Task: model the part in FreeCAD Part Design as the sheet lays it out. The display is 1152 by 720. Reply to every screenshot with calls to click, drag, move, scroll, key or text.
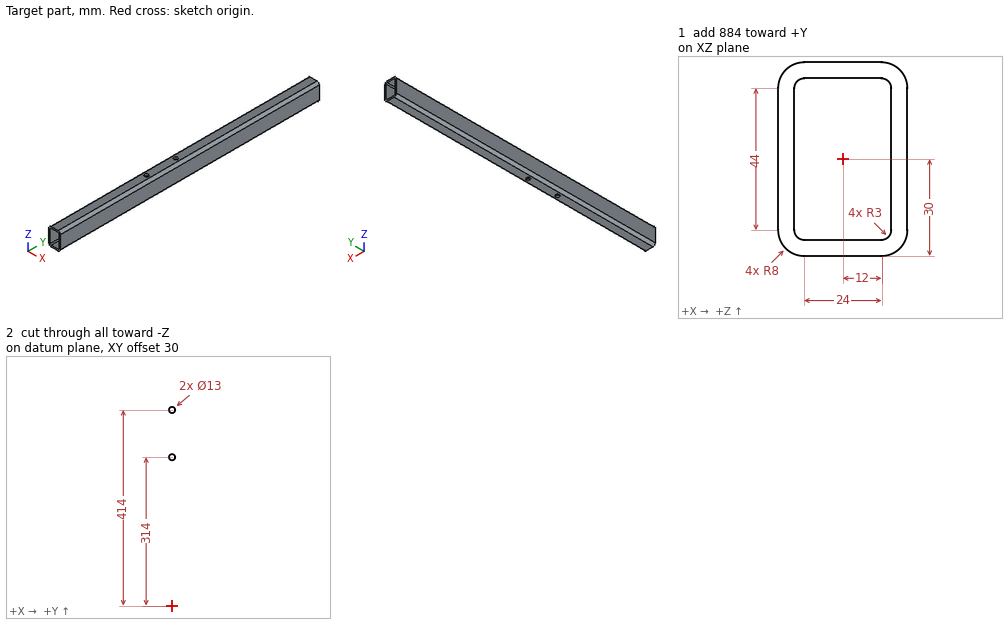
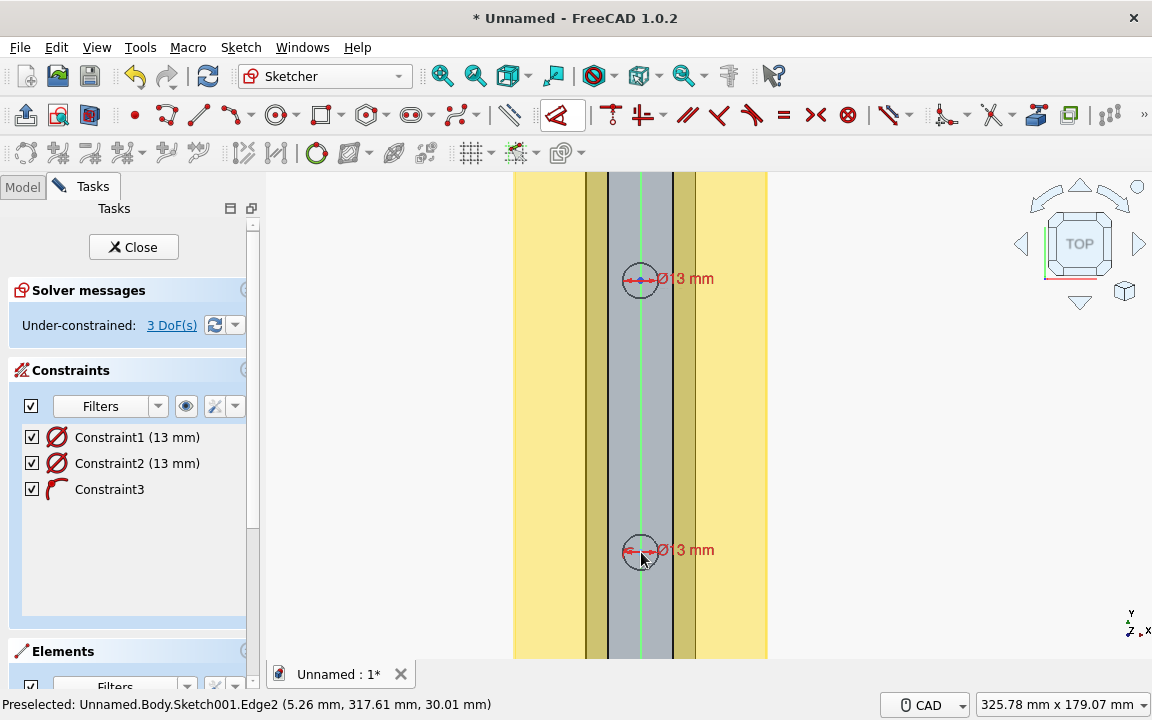
click(640, 281)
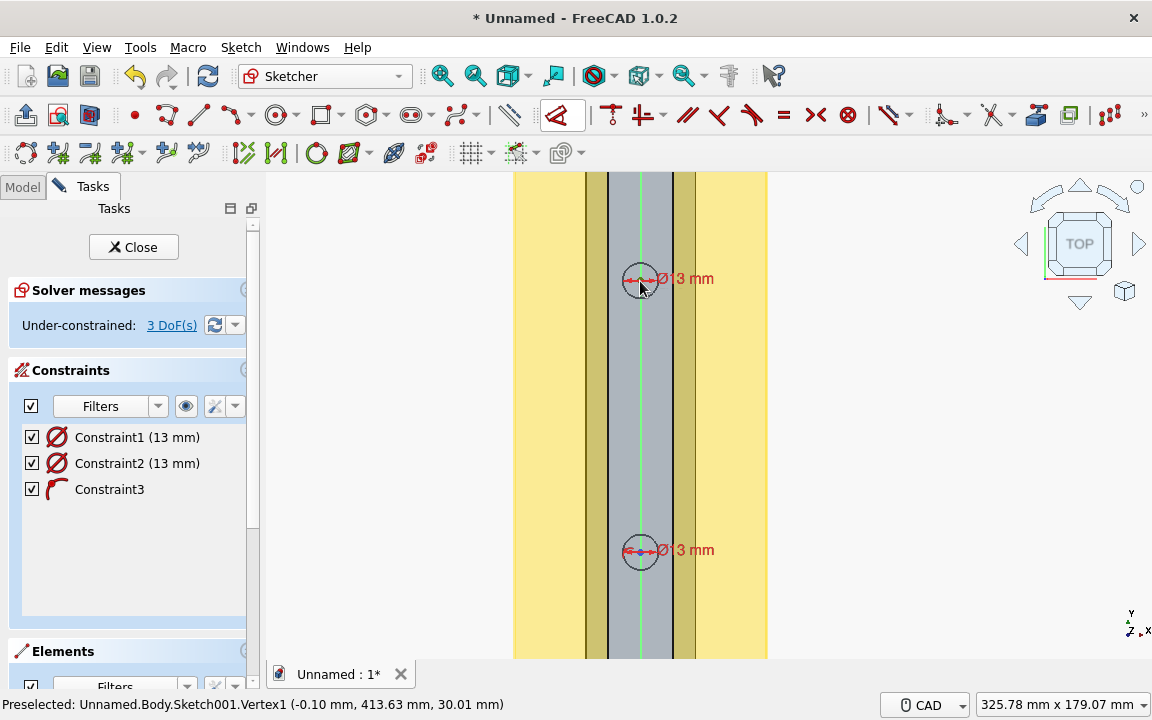
click(641, 600)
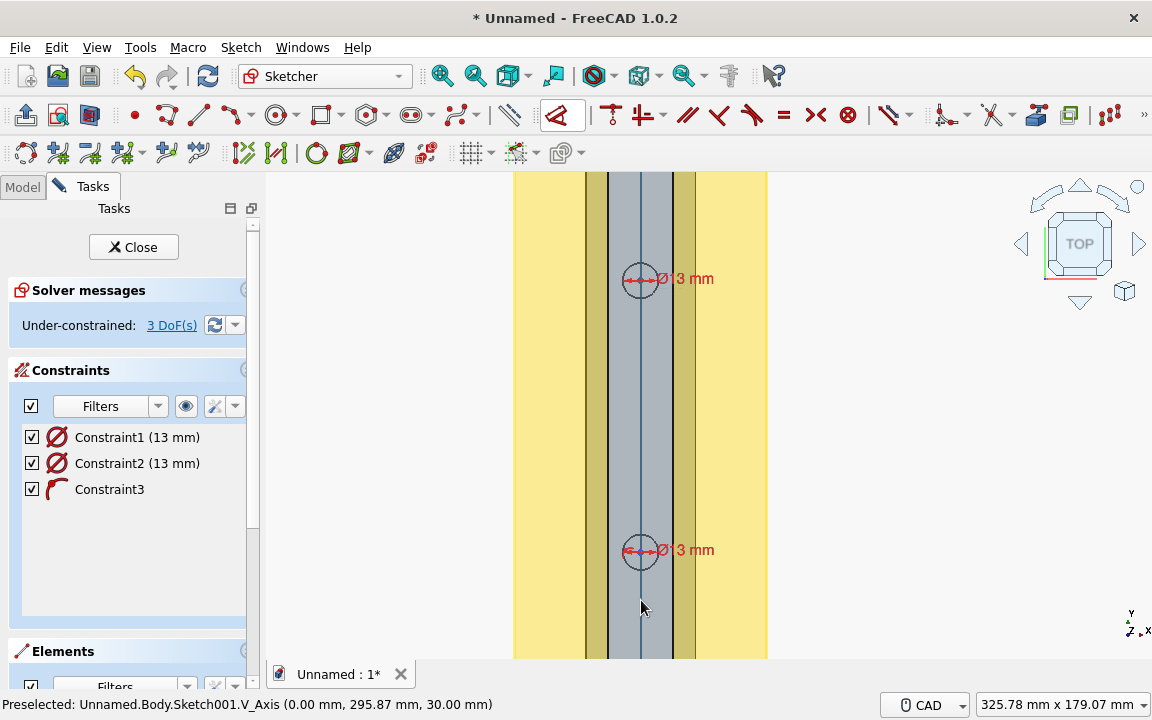
key(c)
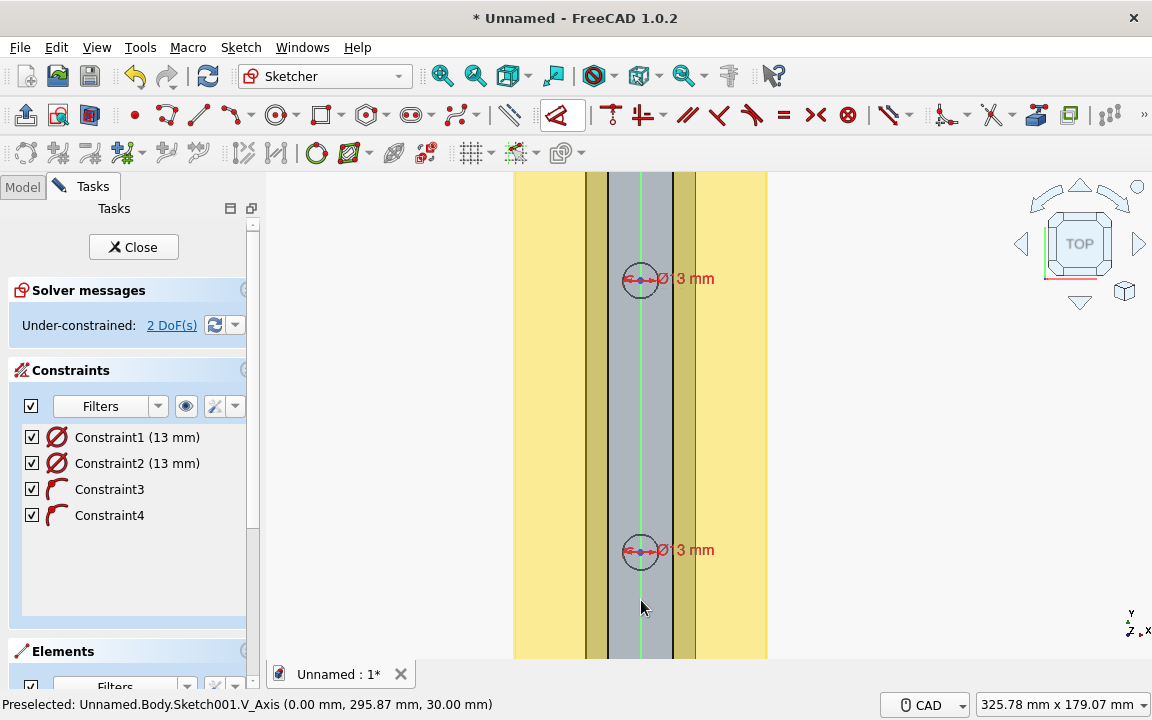
click(641, 281)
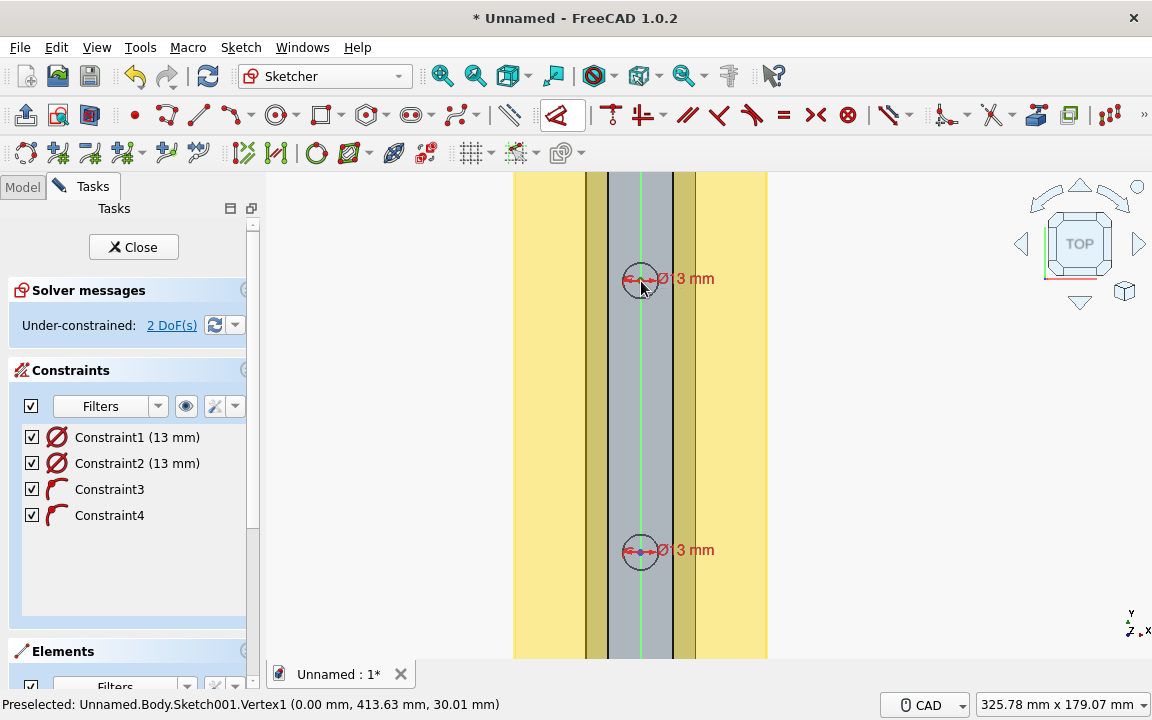
key(i)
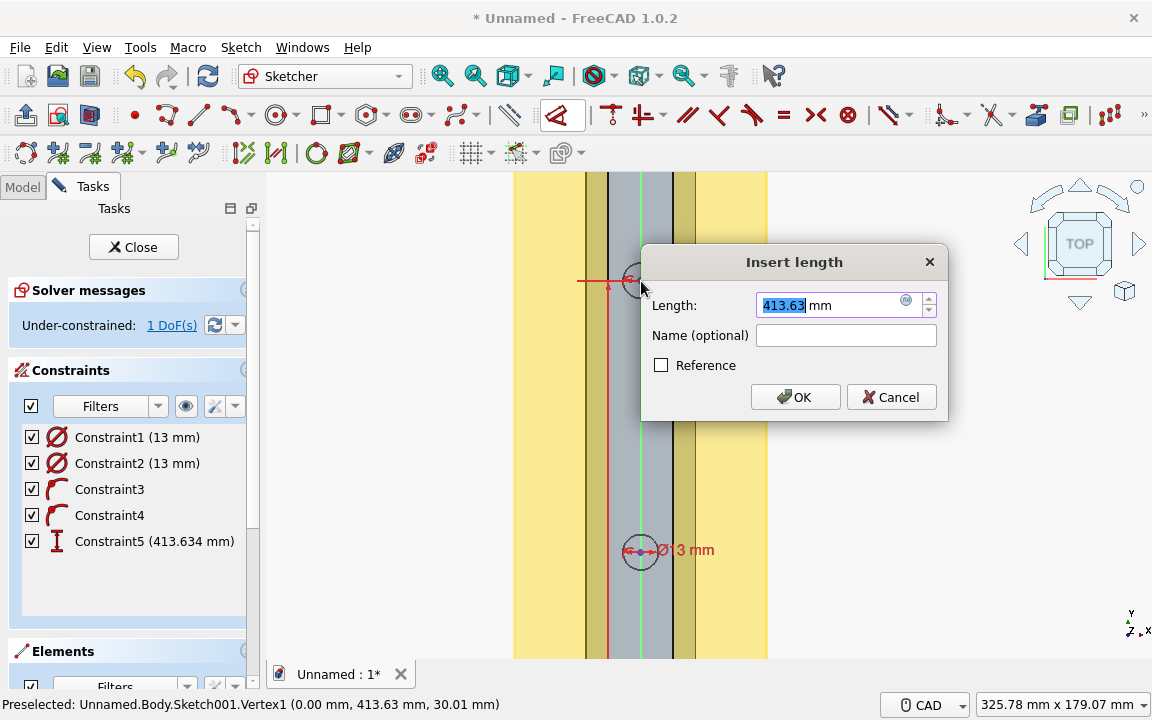
text(414)
key(Return)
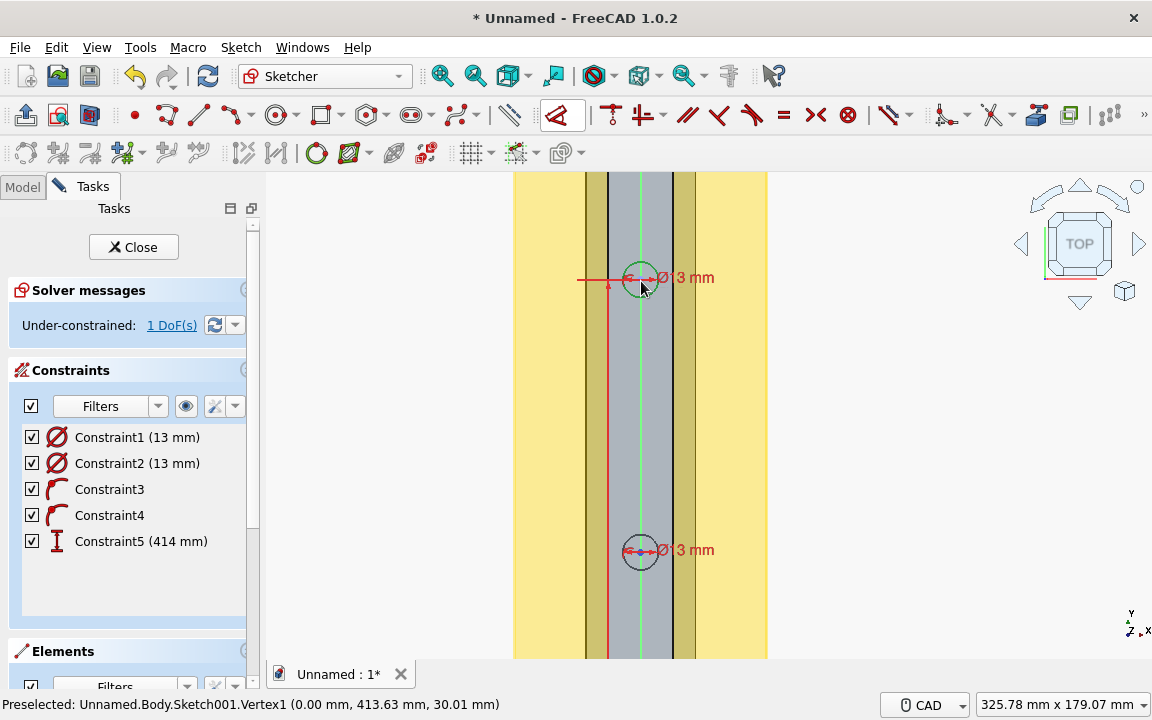
click(641, 552)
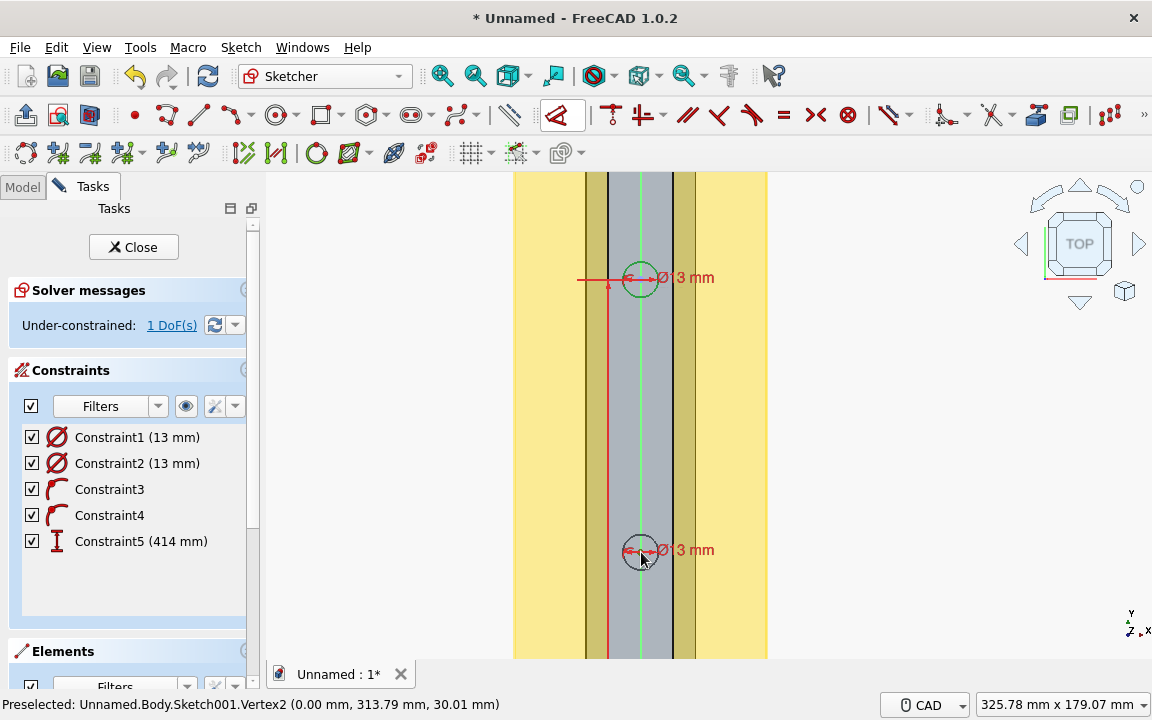
key(i)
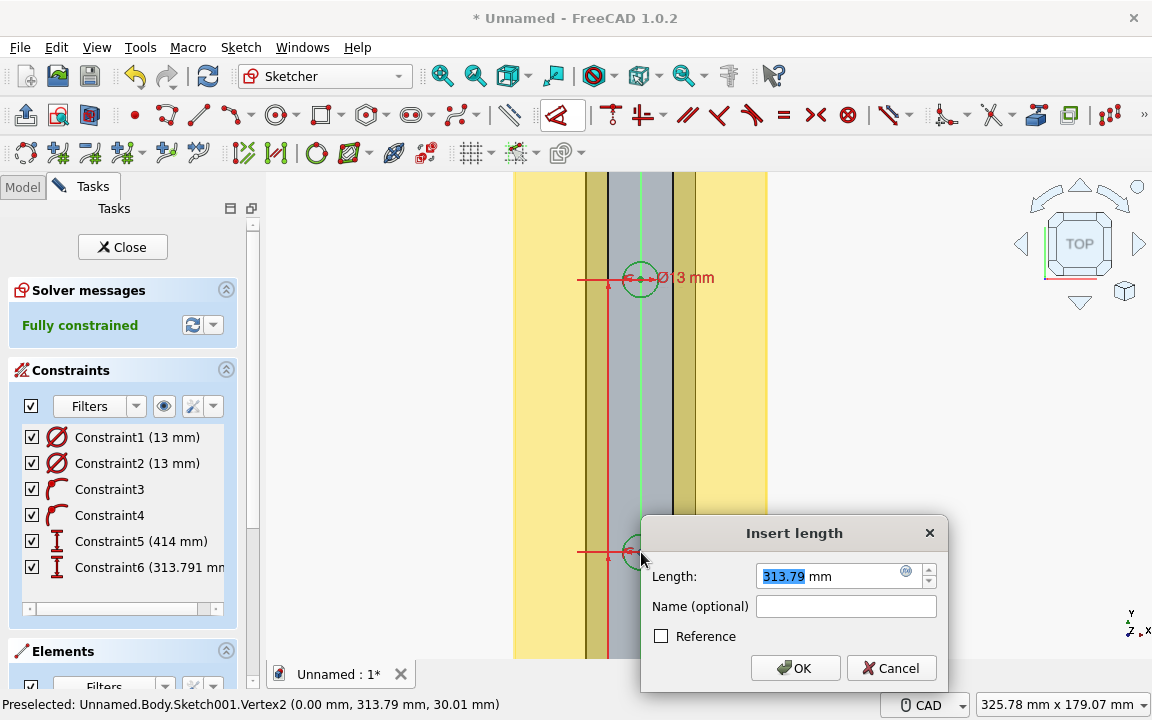
text(314)
key(Return)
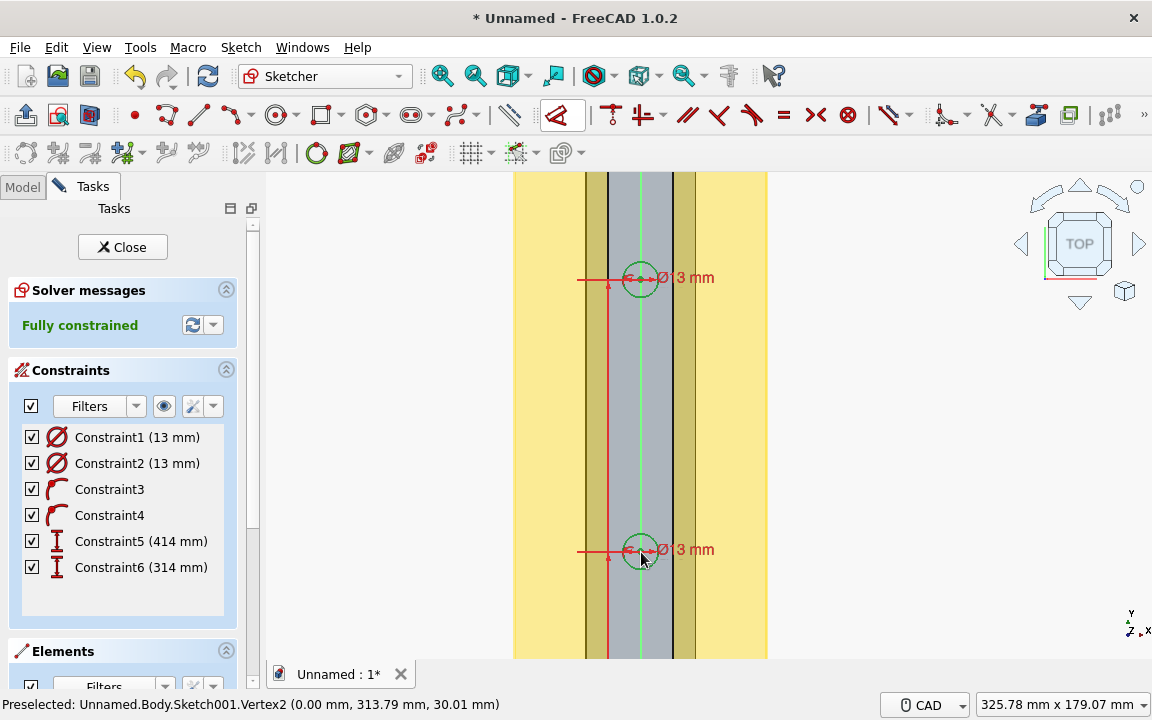
click(123, 247)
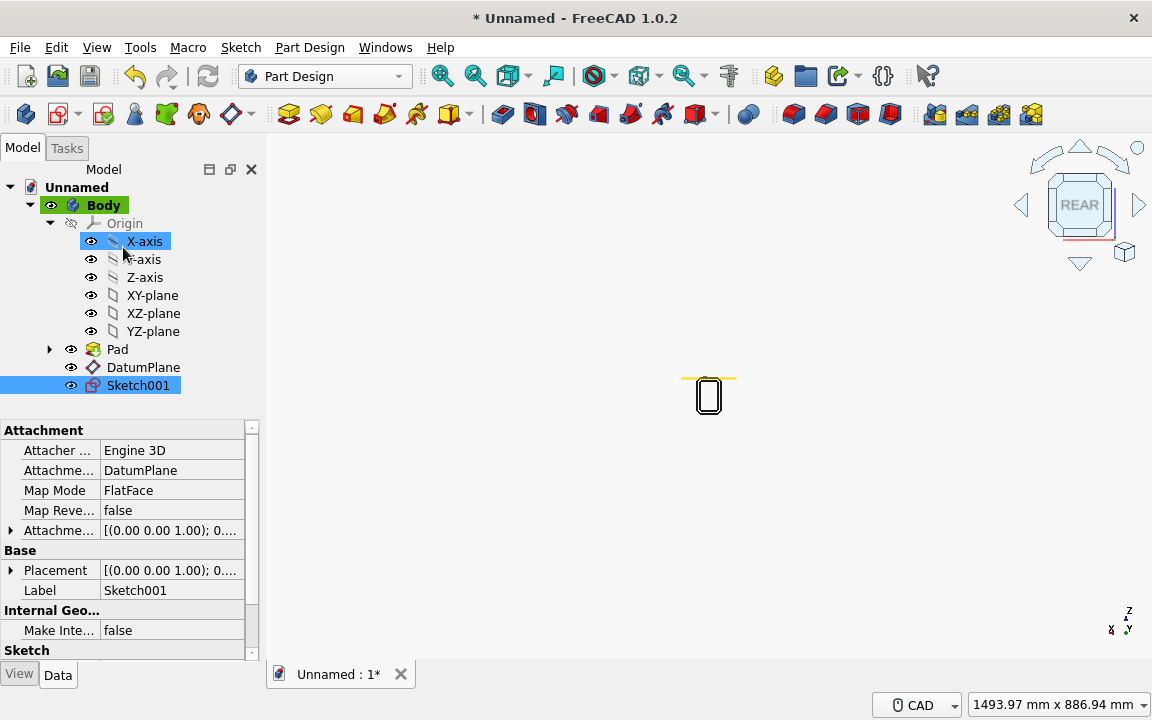
click(504, 114)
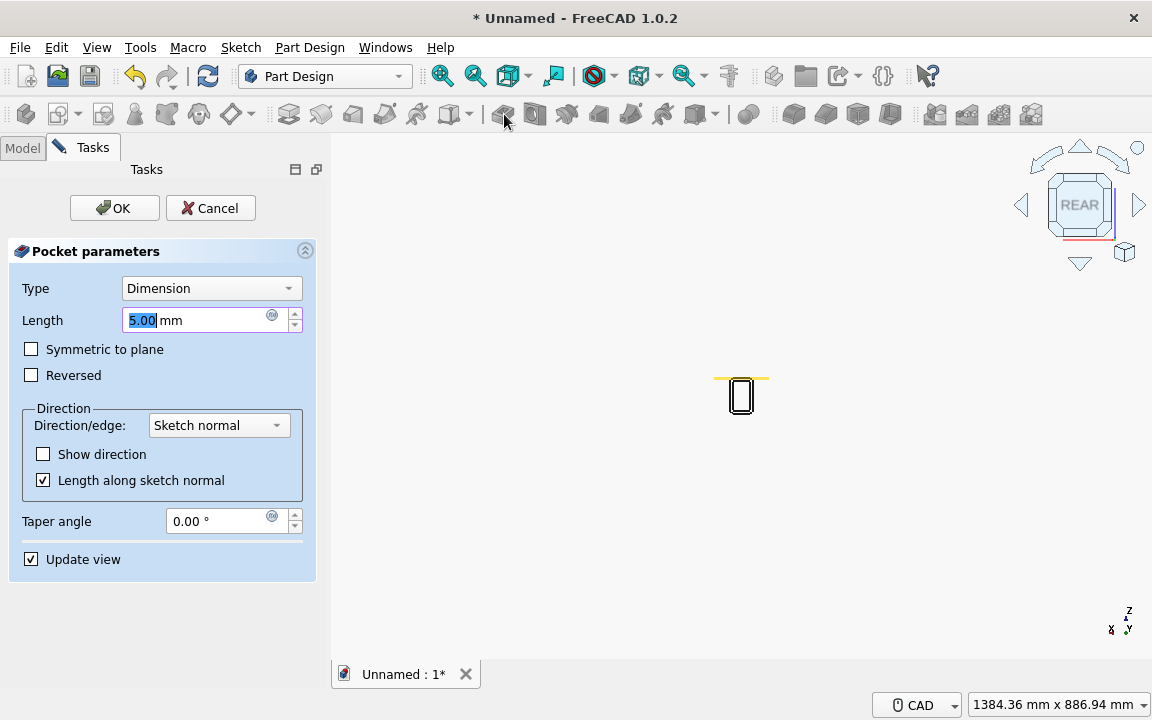
click(212, 288)